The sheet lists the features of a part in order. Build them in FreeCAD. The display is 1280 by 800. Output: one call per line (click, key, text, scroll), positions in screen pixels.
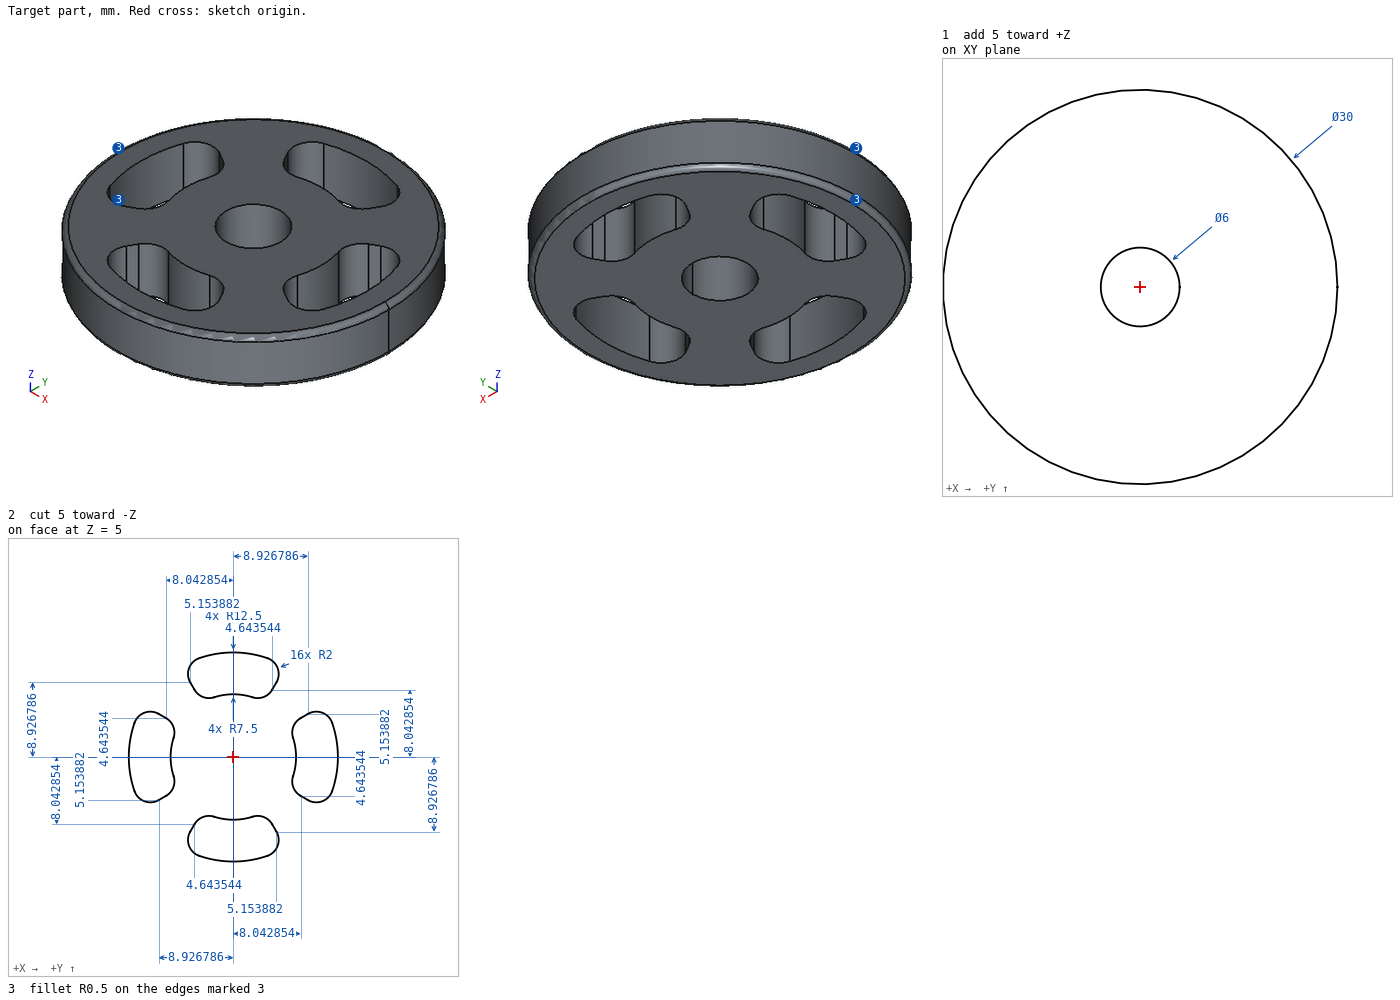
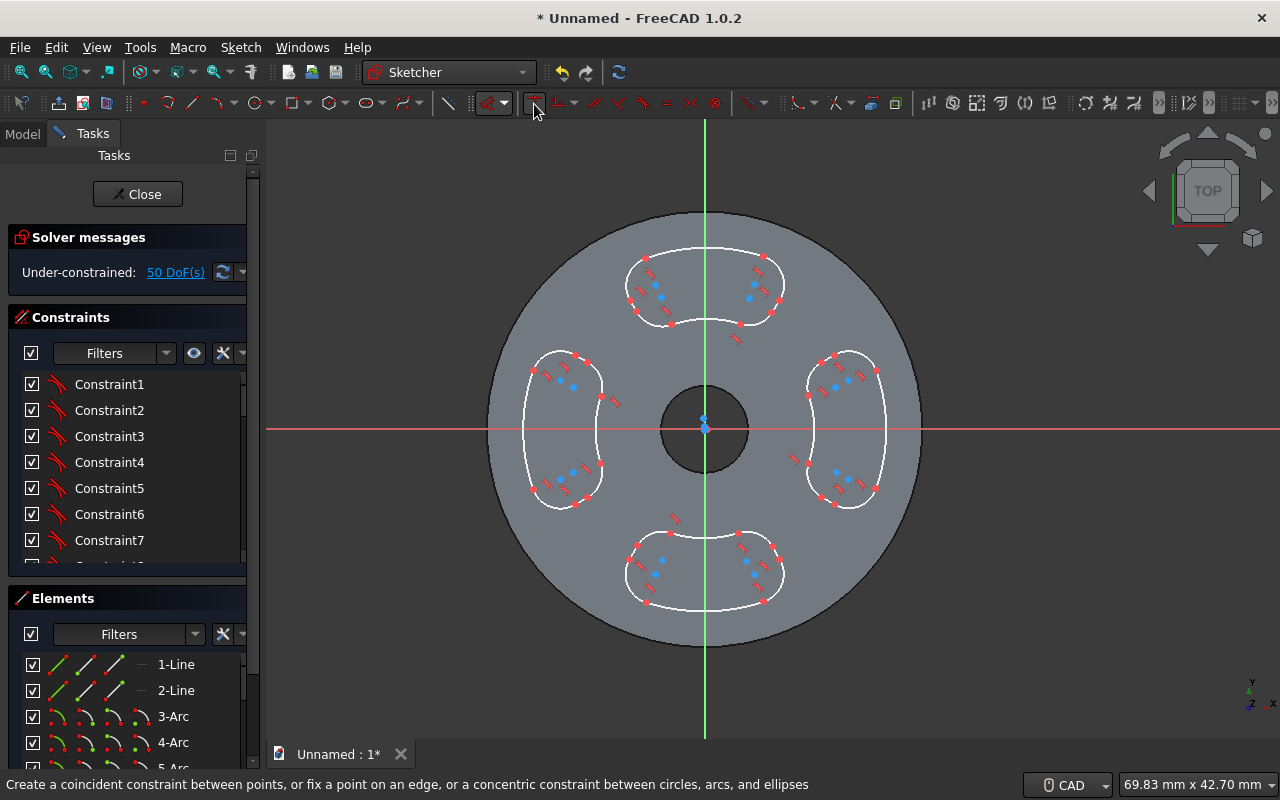
click(720, 320)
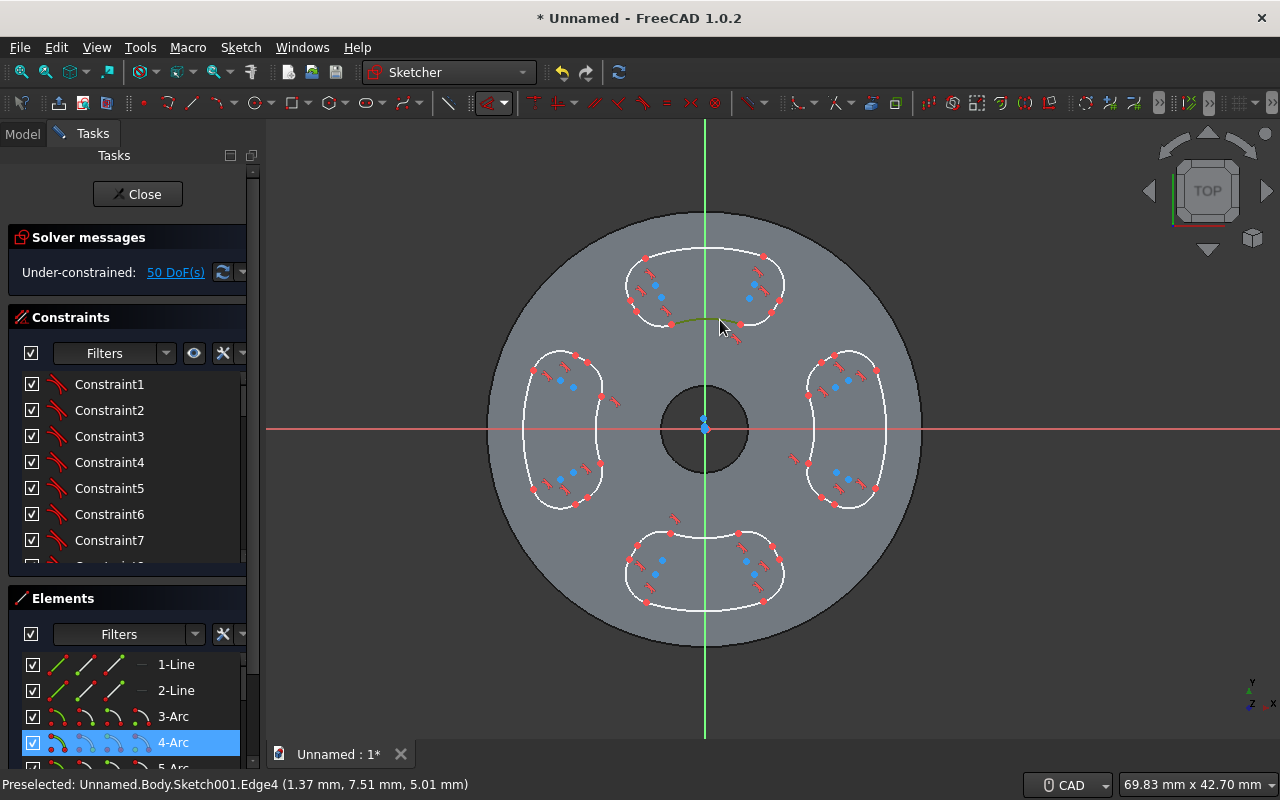
click(691, 537)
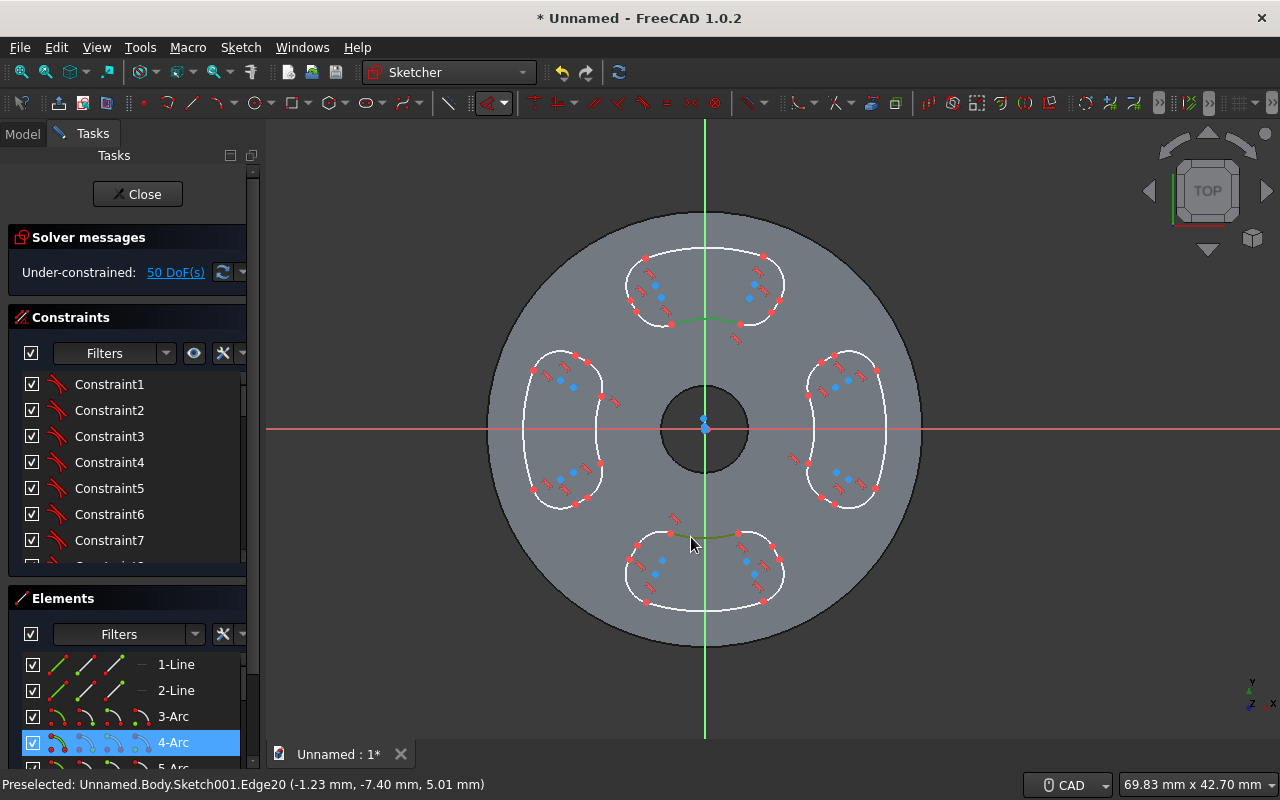
click(534, 104)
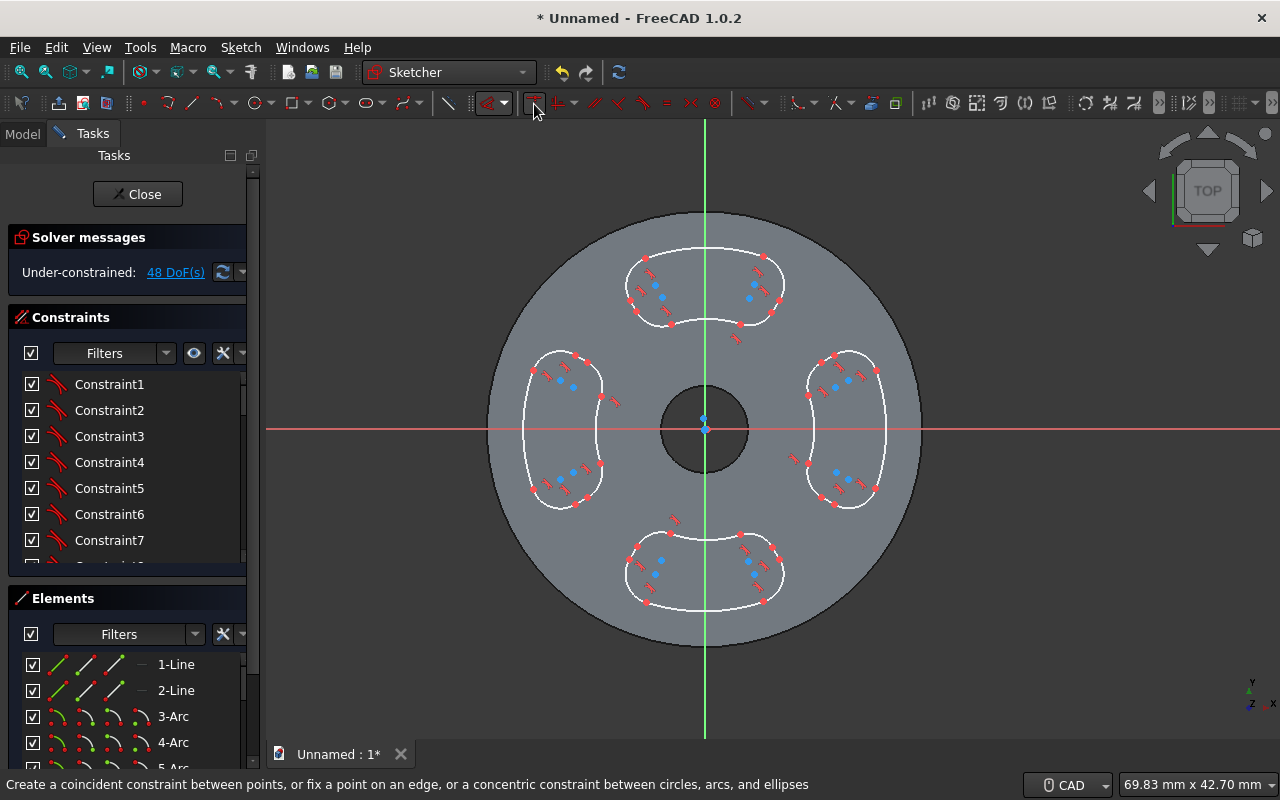
click(720, 320)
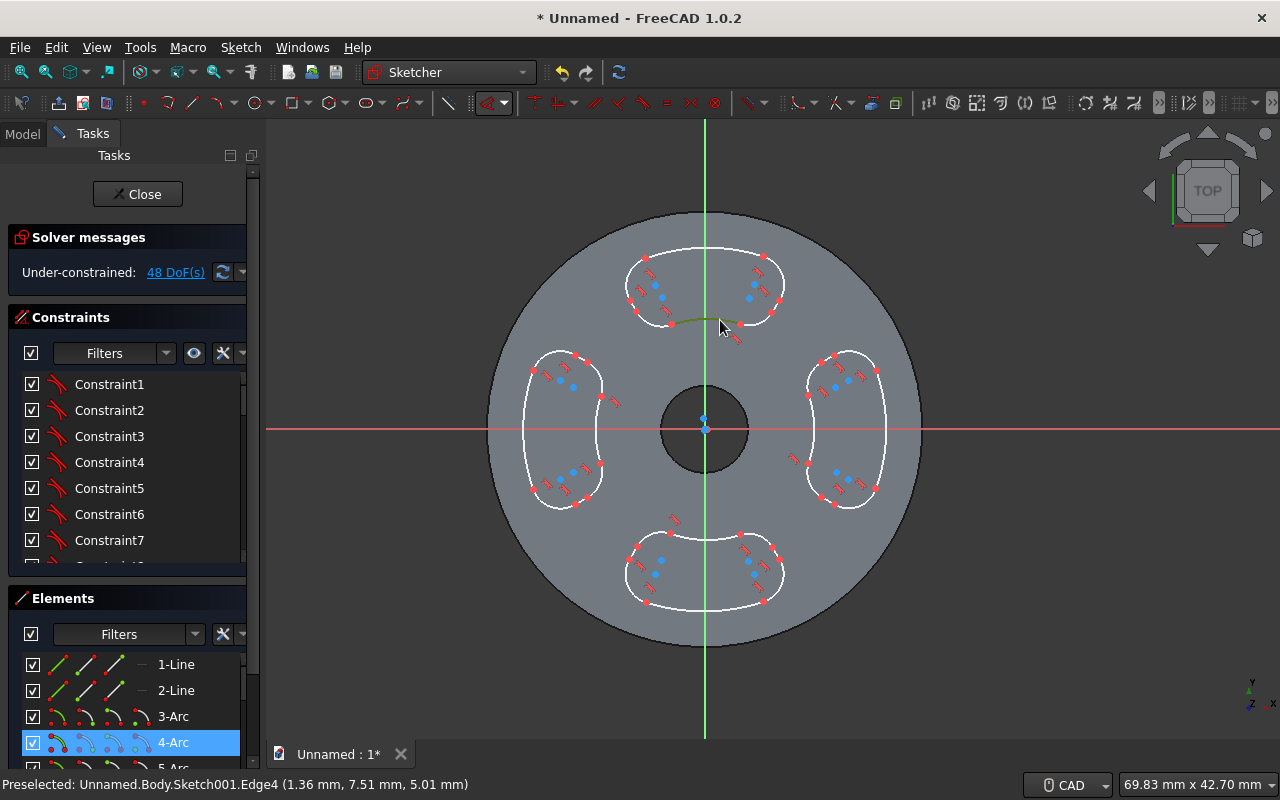
click(681, 610)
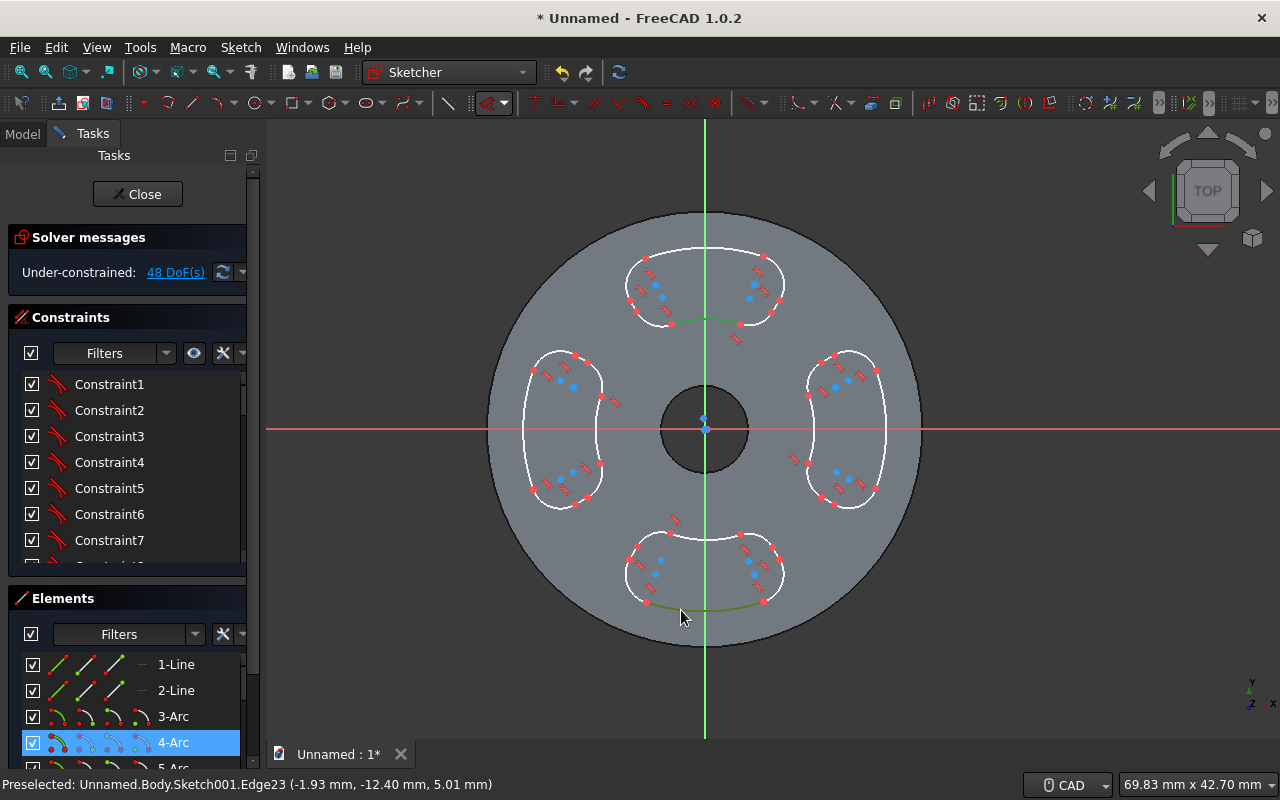
click(534, 104)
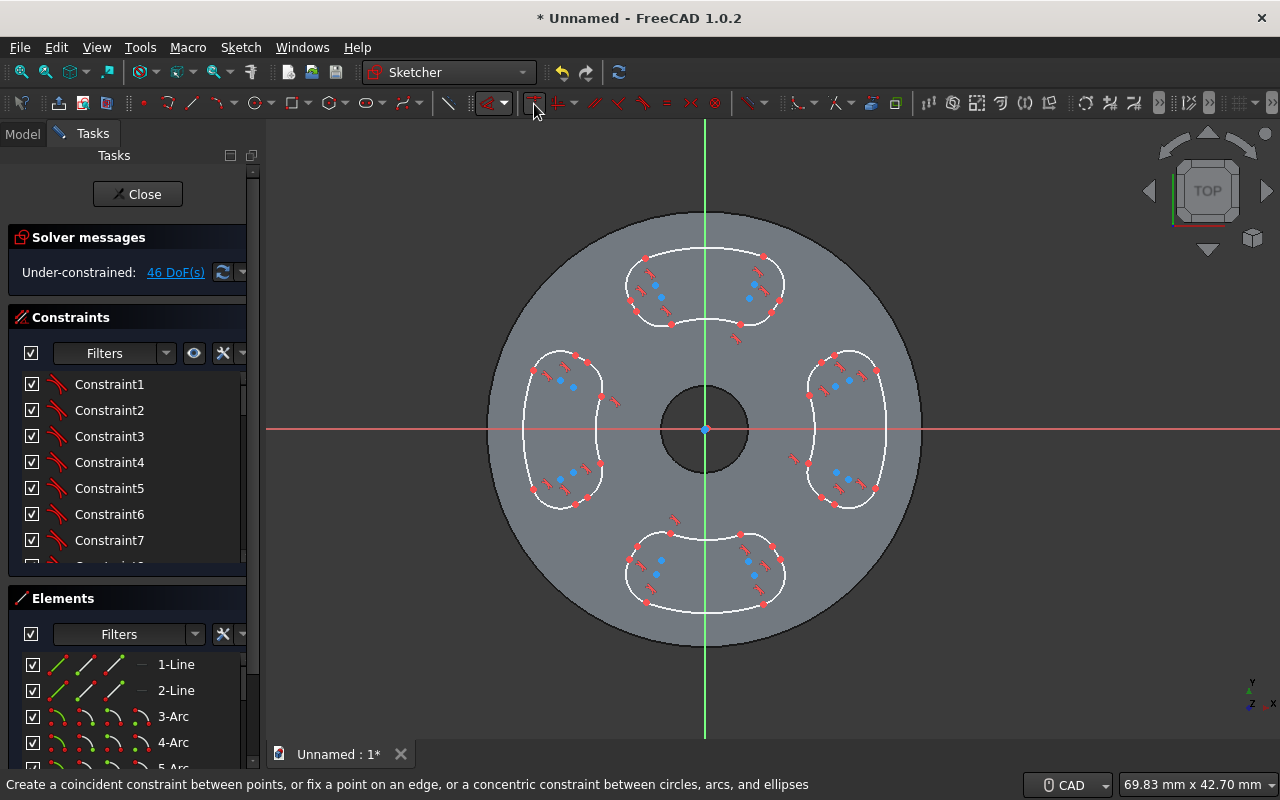
click(720, 320)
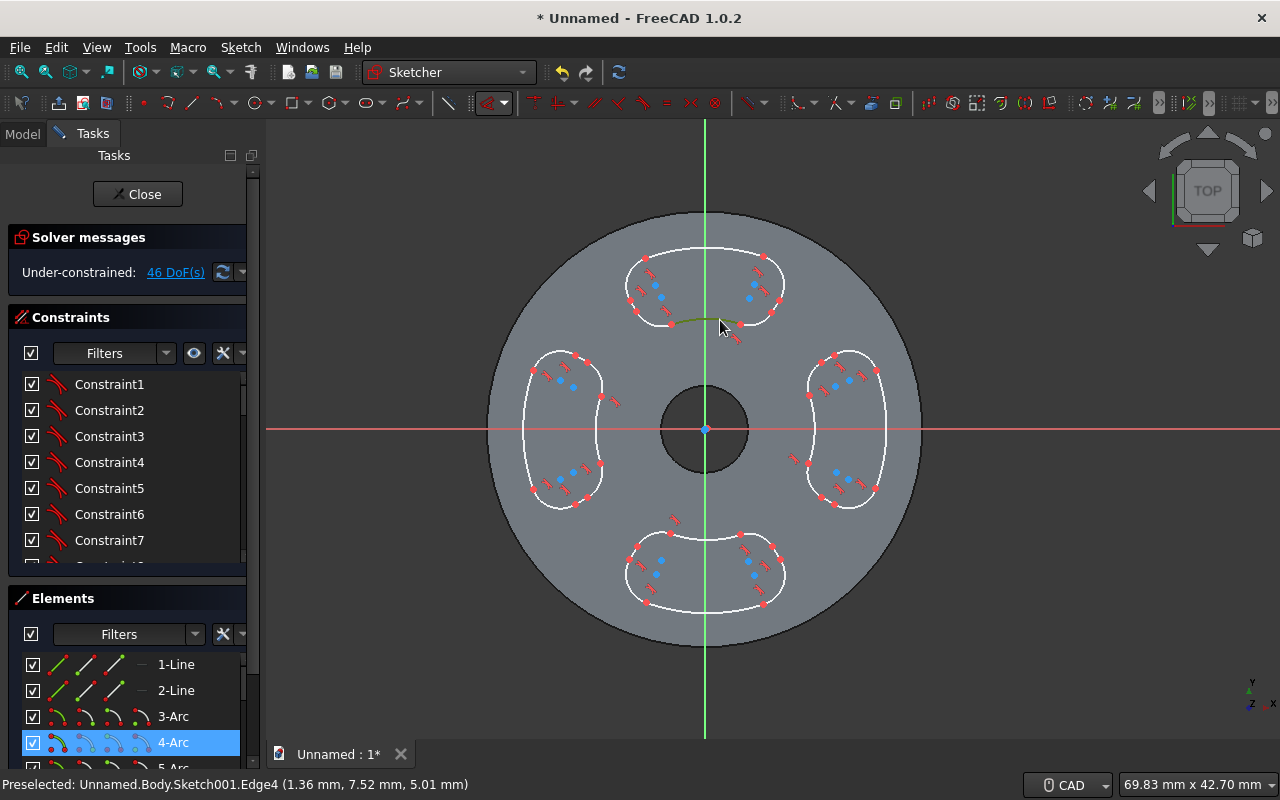
click(597, 416)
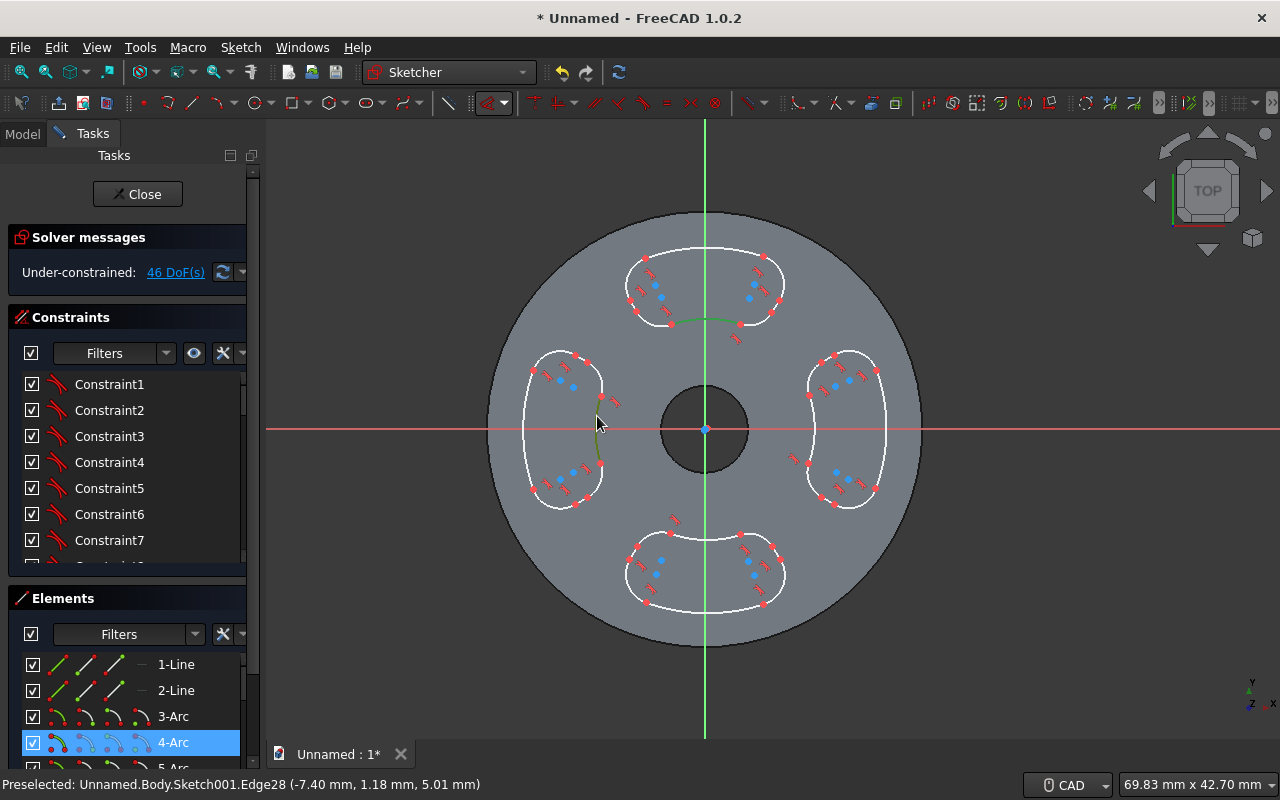
click(534, 104)